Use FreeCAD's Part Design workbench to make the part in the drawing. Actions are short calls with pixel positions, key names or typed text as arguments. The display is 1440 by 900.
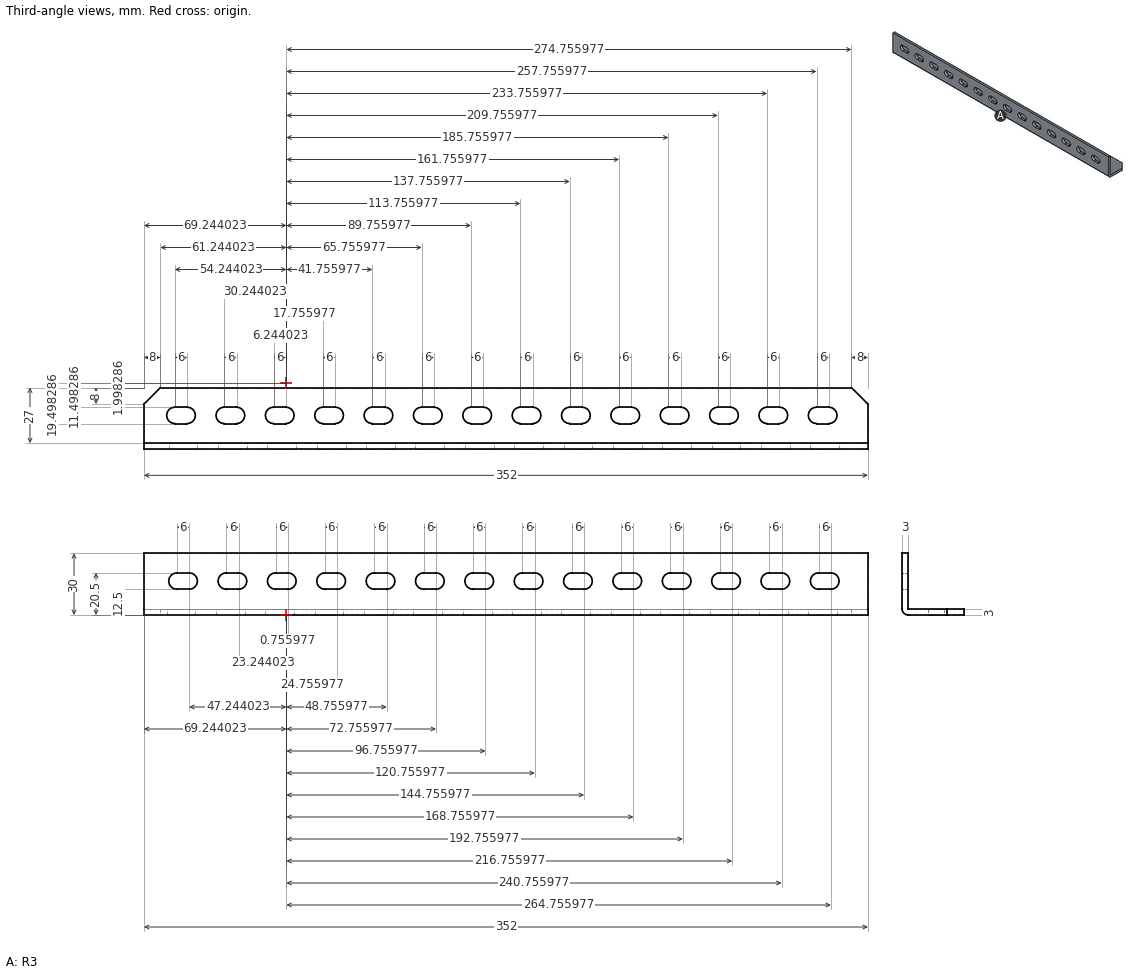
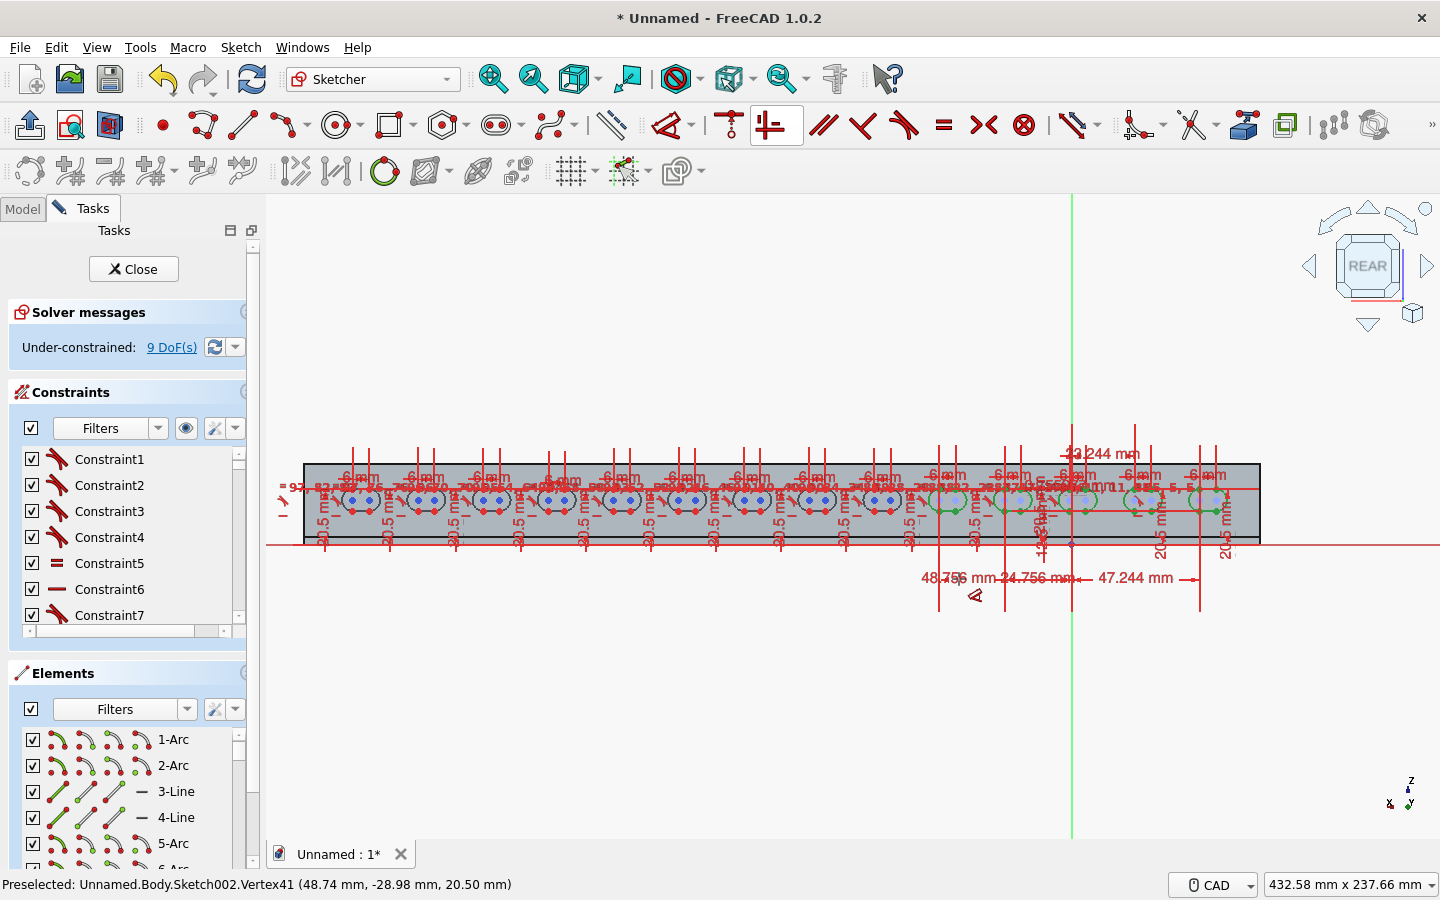
click(874, 489)
click(973, 455)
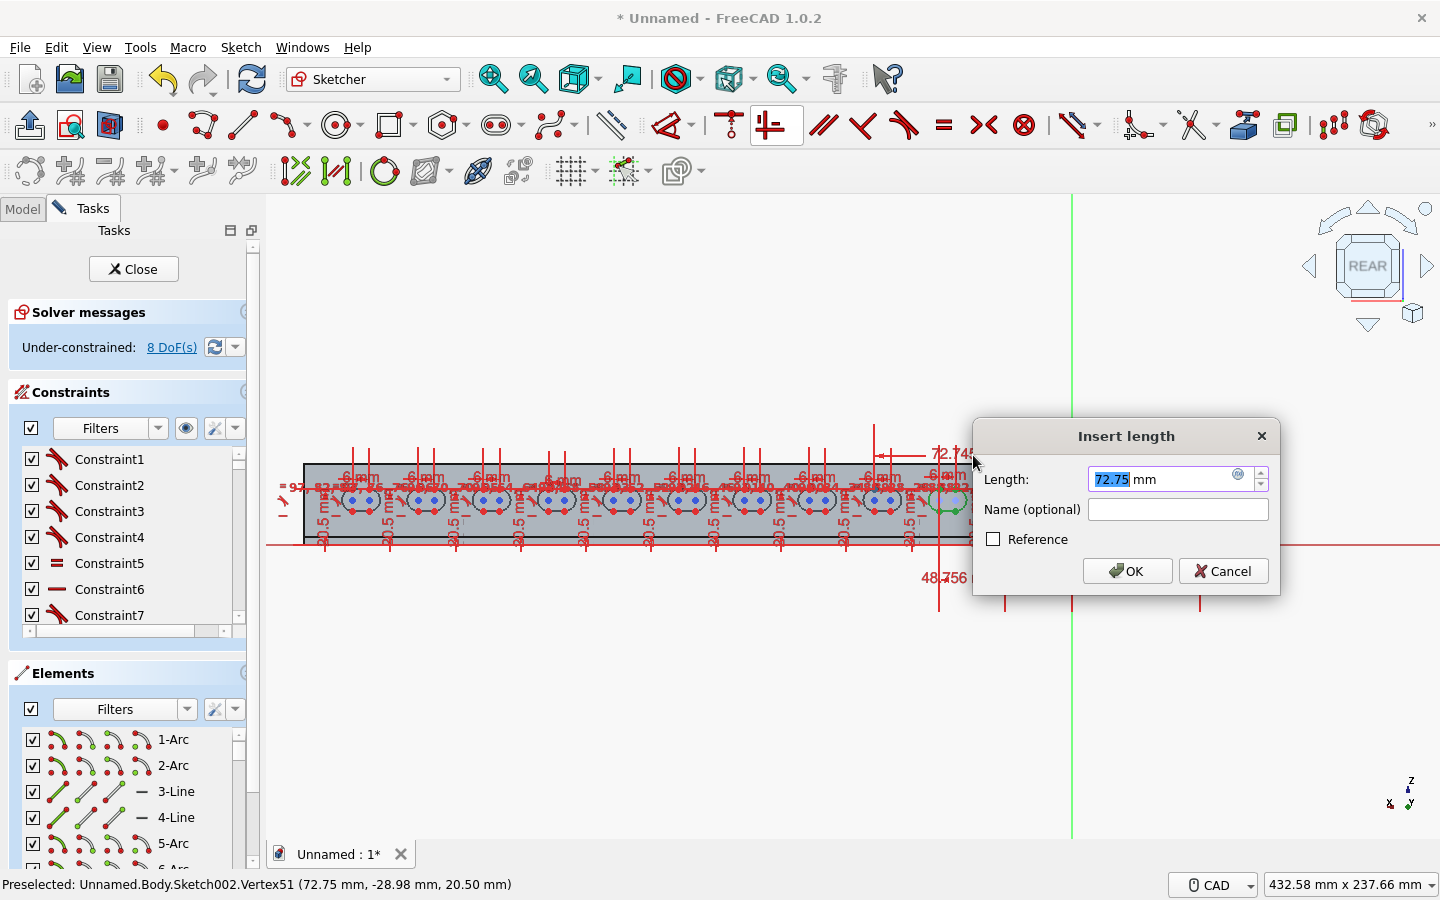
text(72.755977)
key(Return)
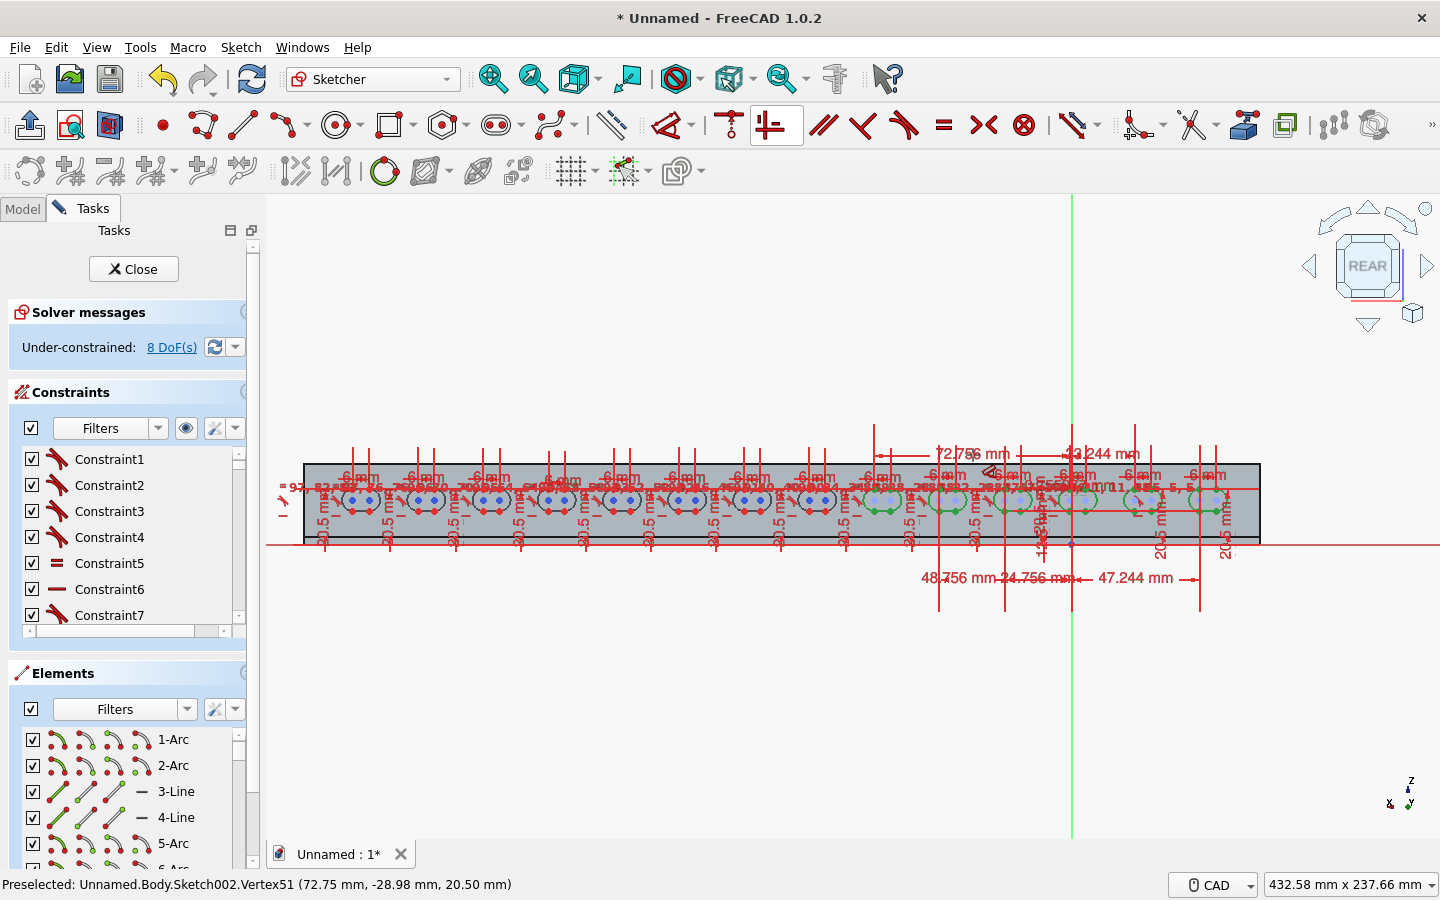
click(809, 489)
click(880, 579)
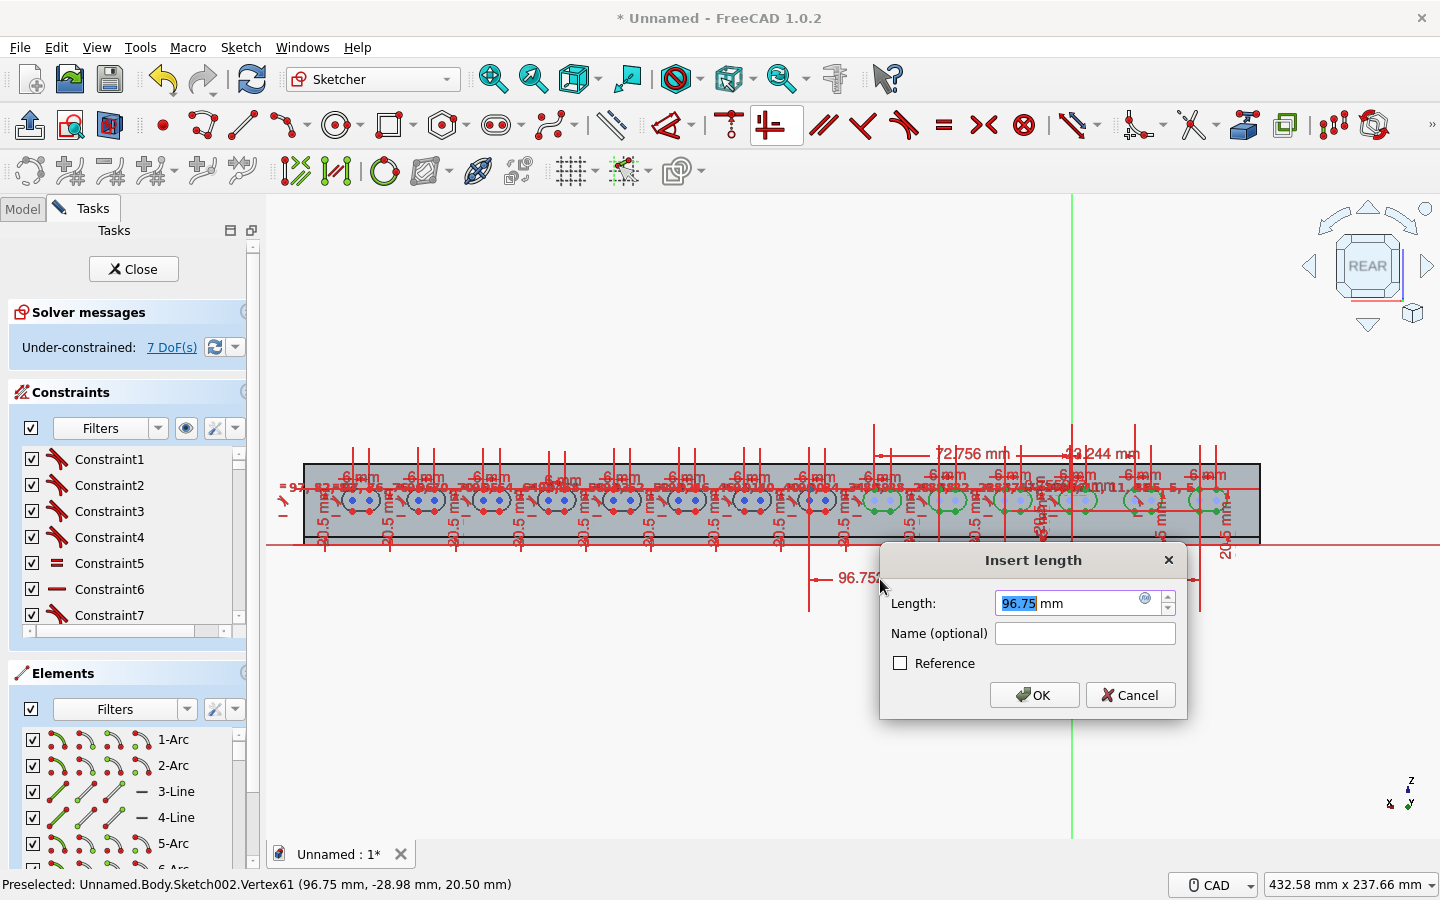
text(96.755977)
key(Return)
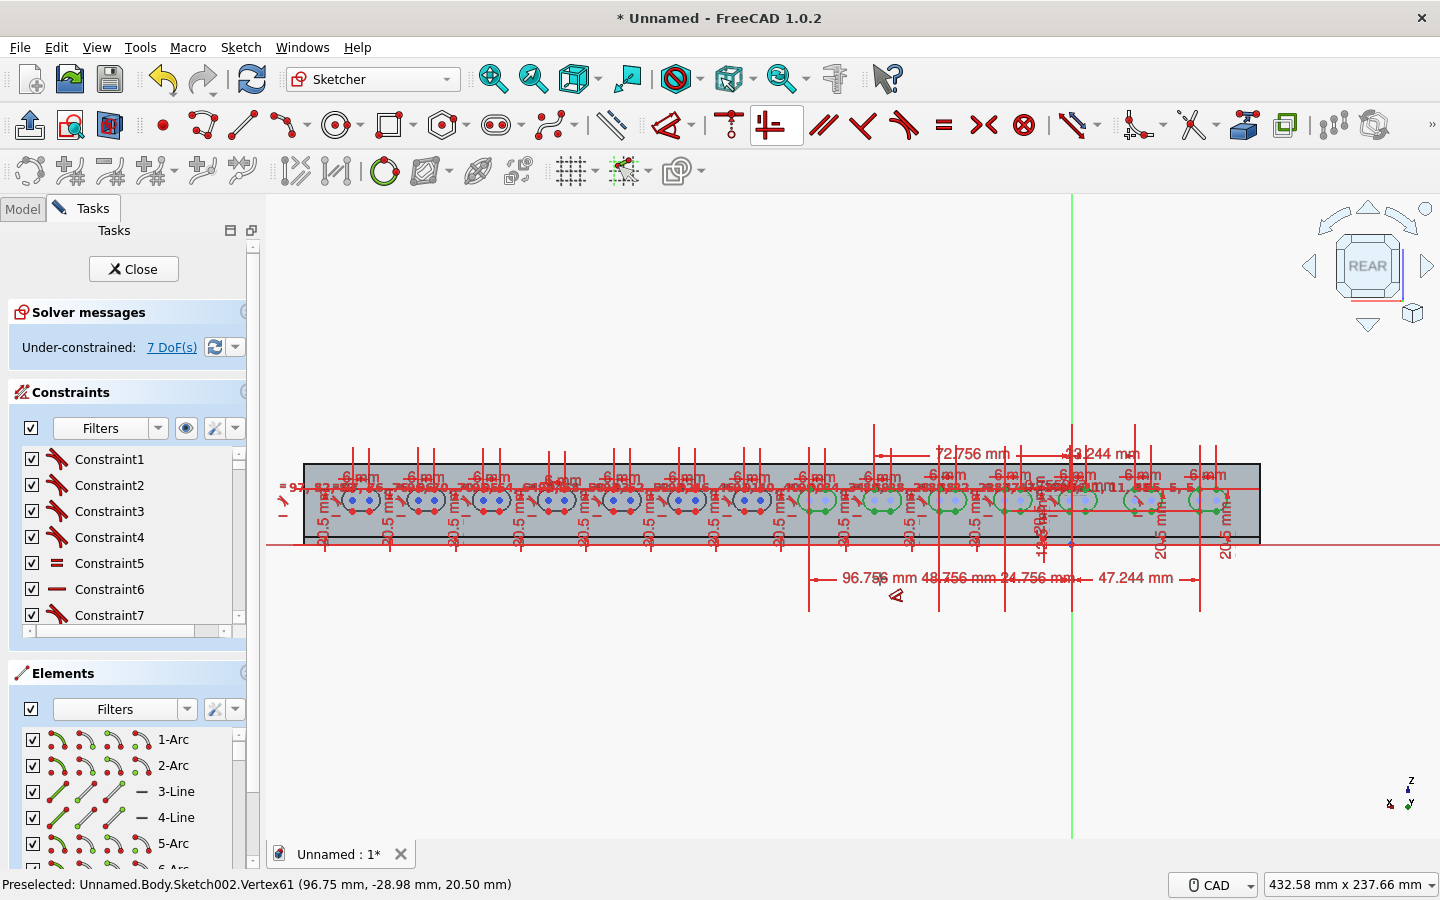
click(744, 489)
click(793, 579)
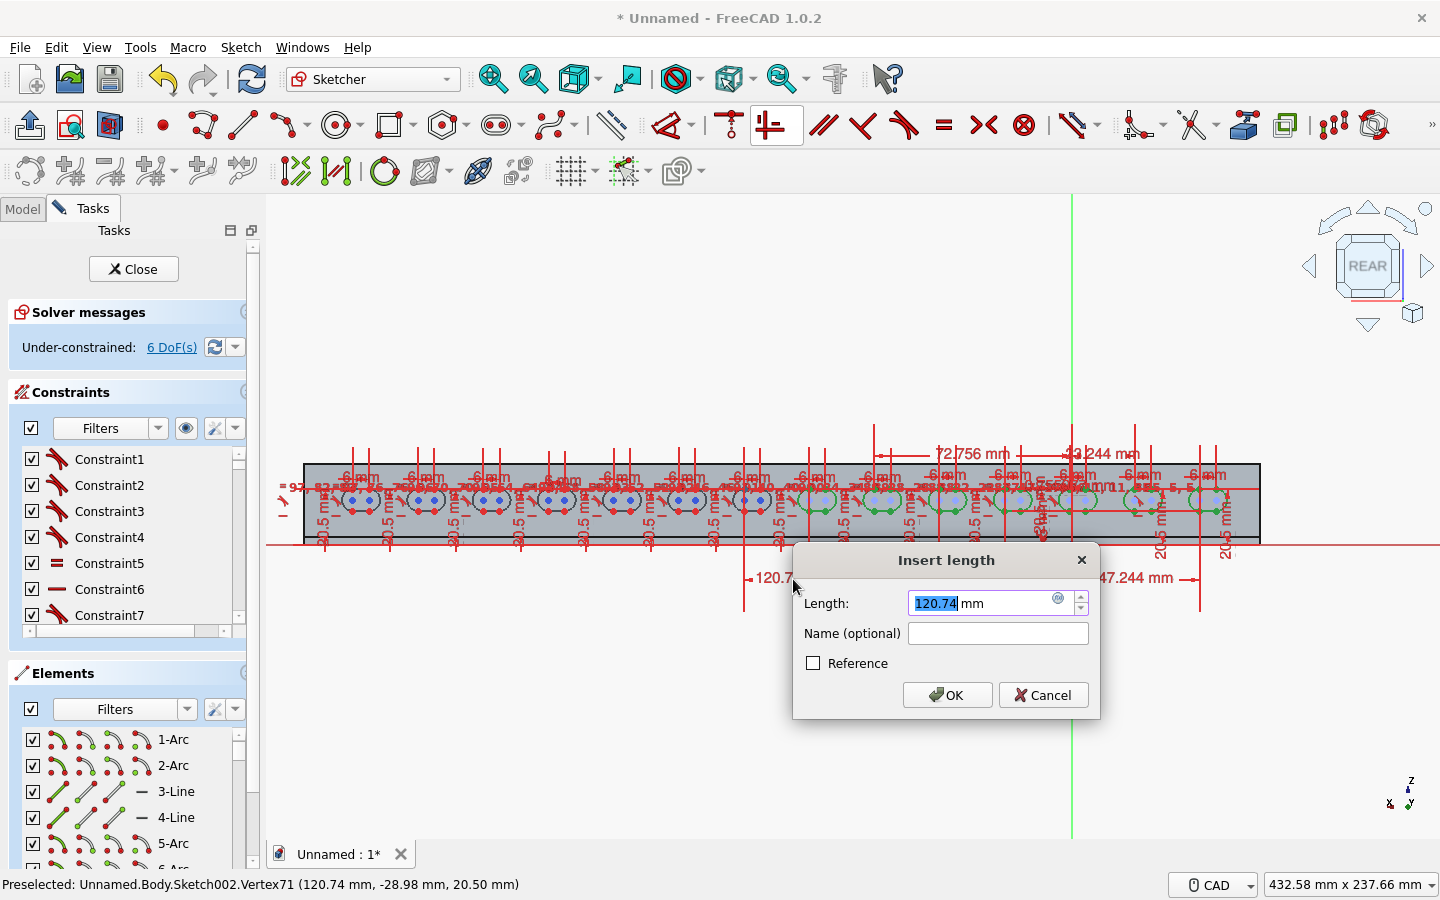
text(120.755977)
key(Return)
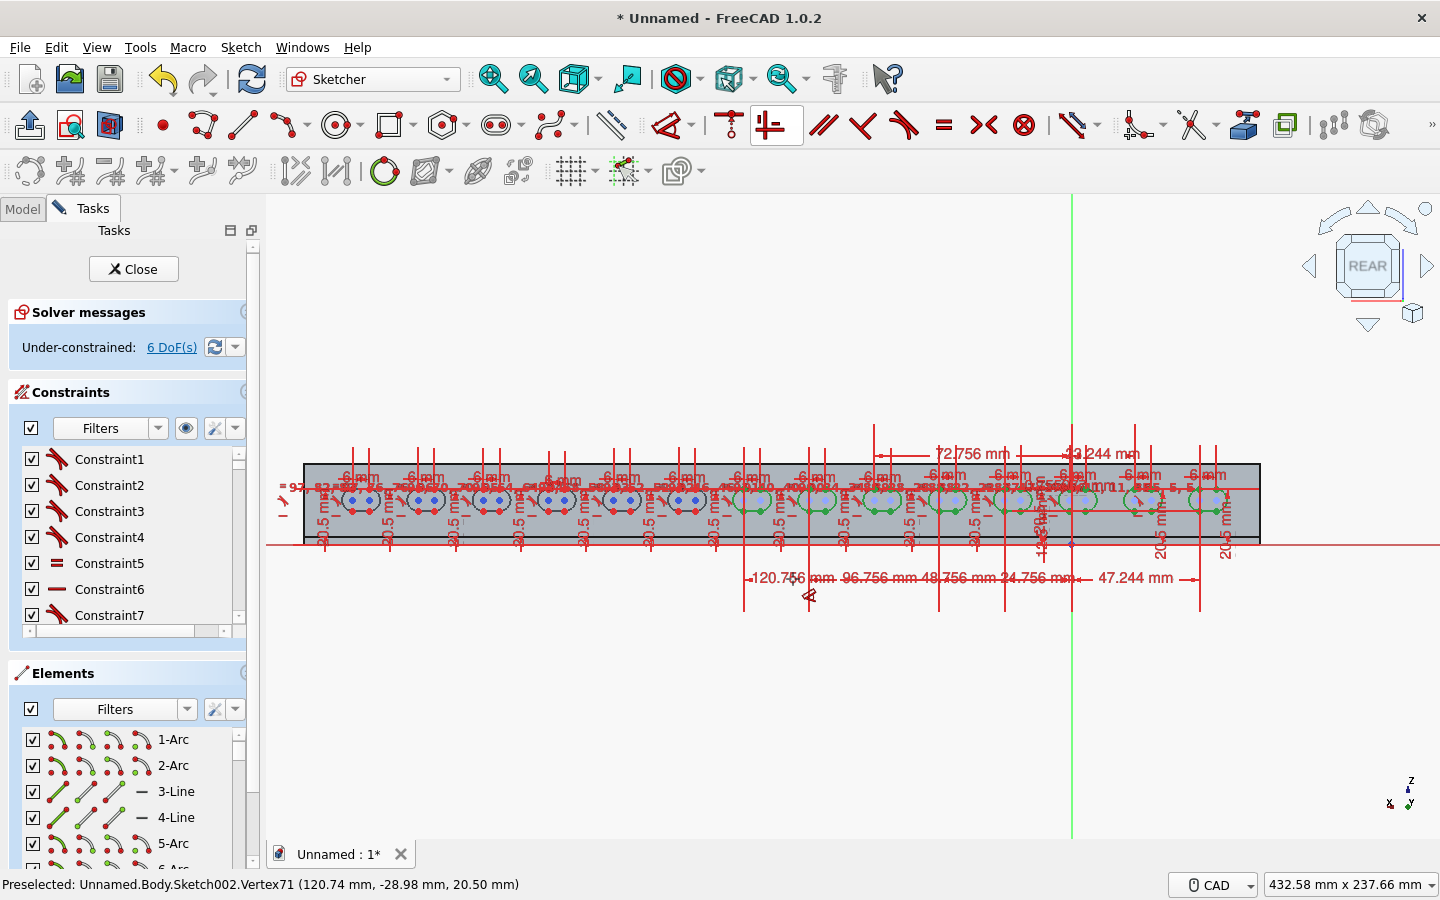
click(679, 489)
click(875, 455)